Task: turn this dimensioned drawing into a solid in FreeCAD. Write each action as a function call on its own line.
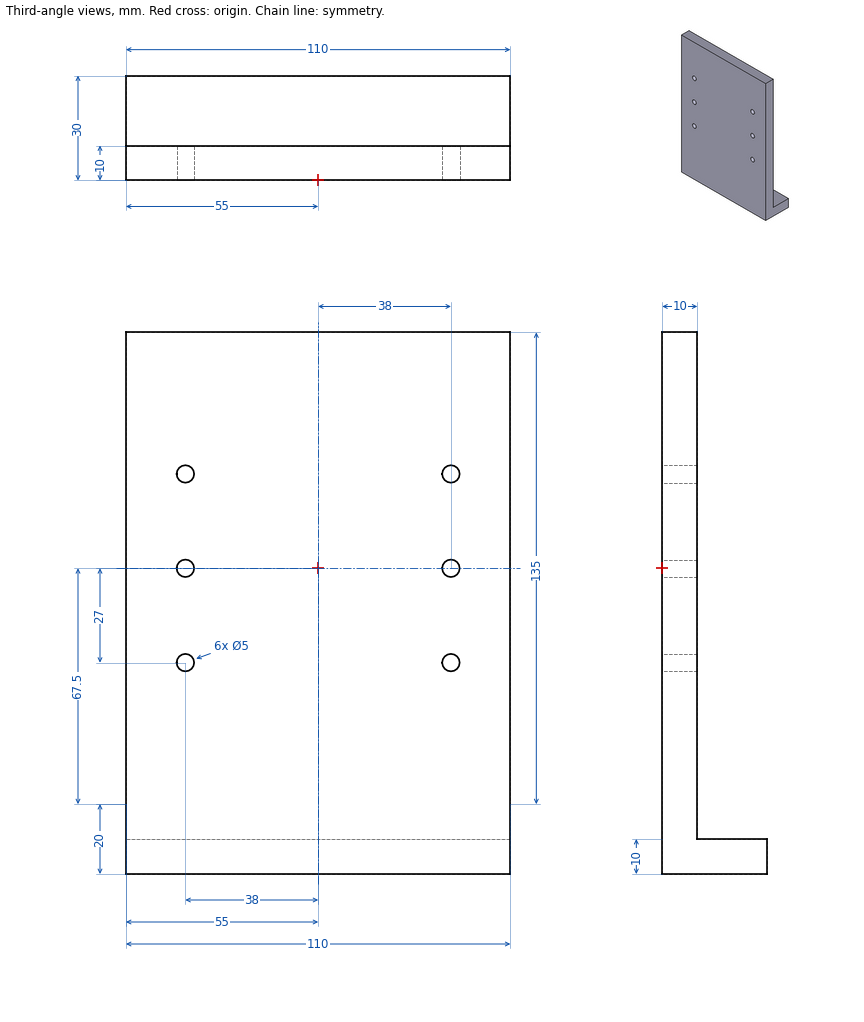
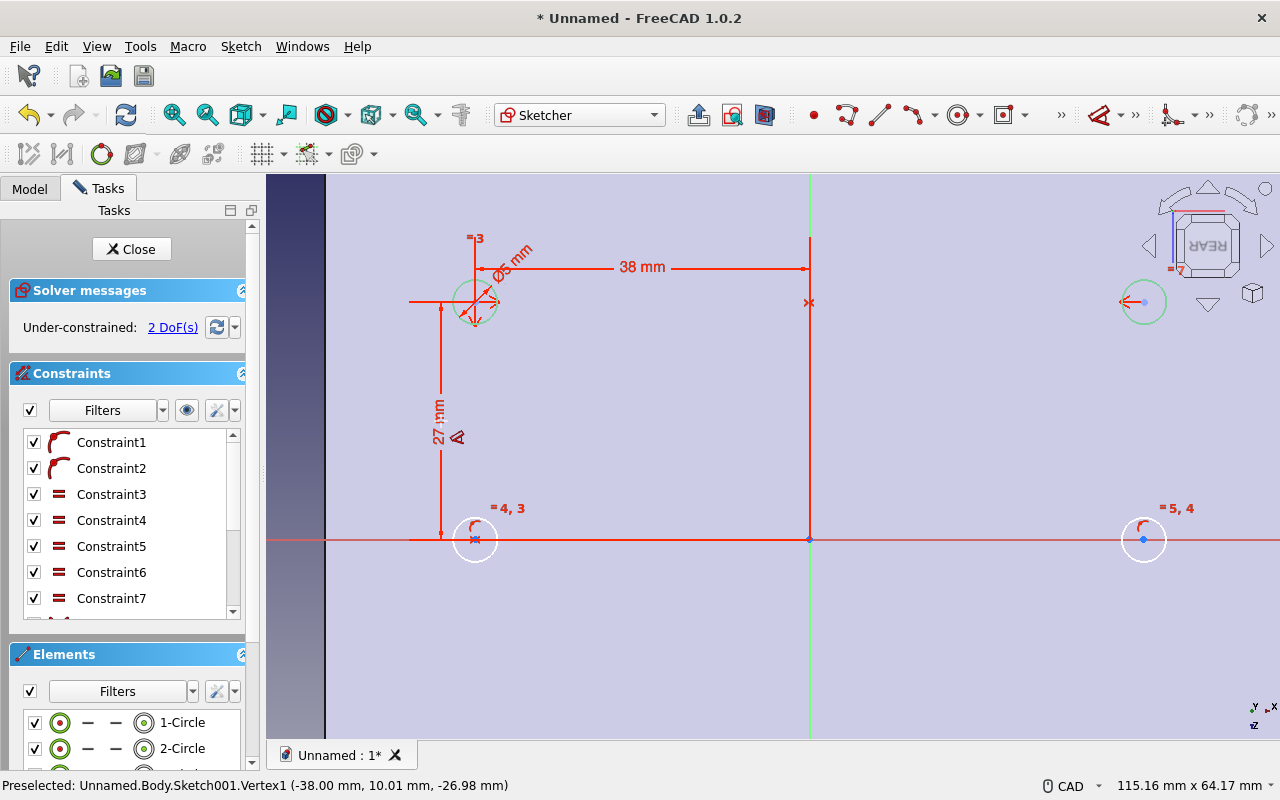
click(475, 540)
click(643, 574)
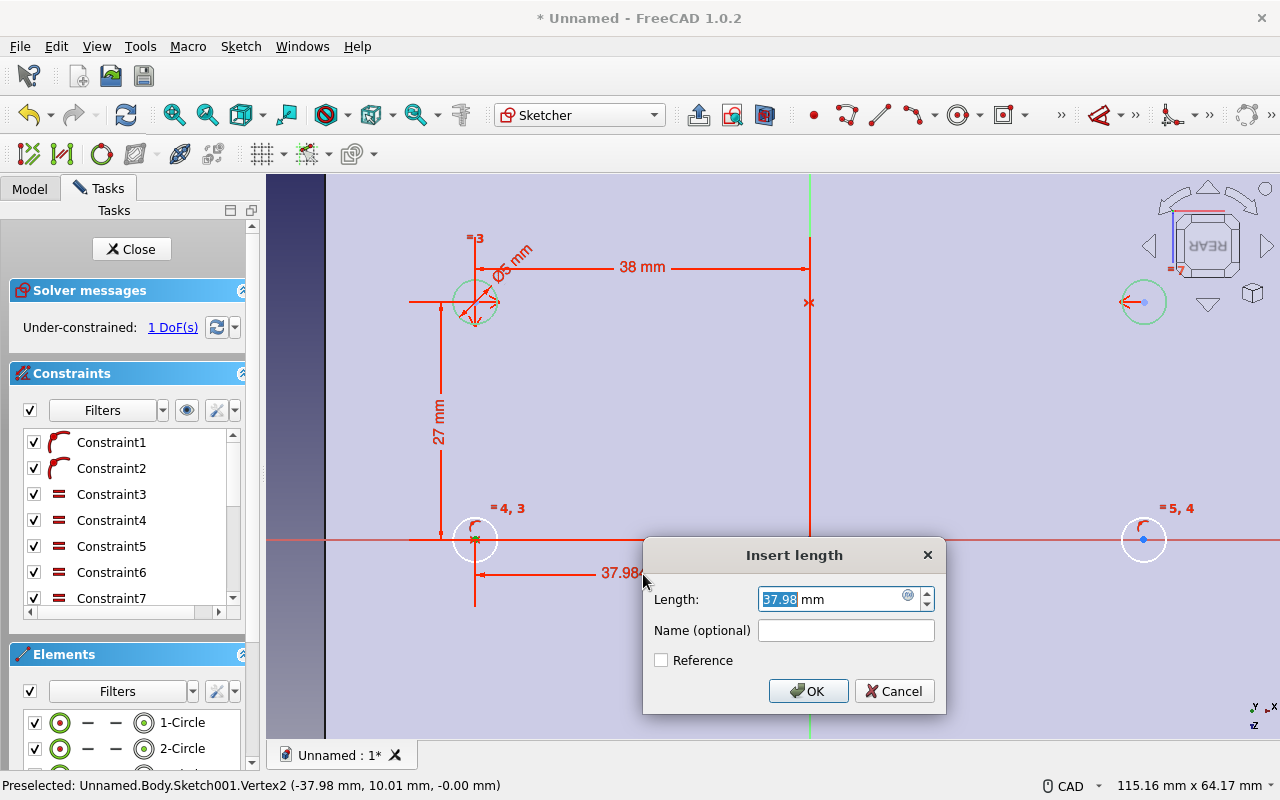
text(38)
key(Return)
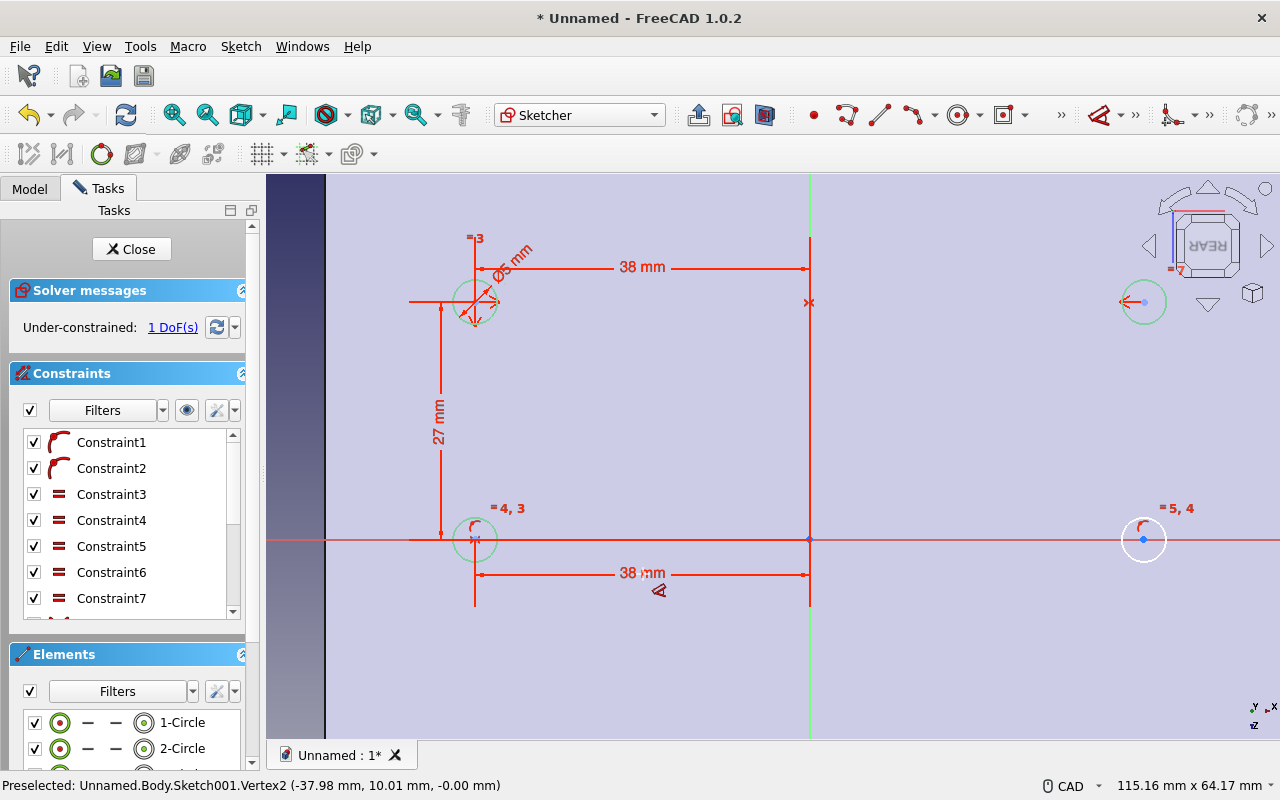
scroll(491, 287, down, 2)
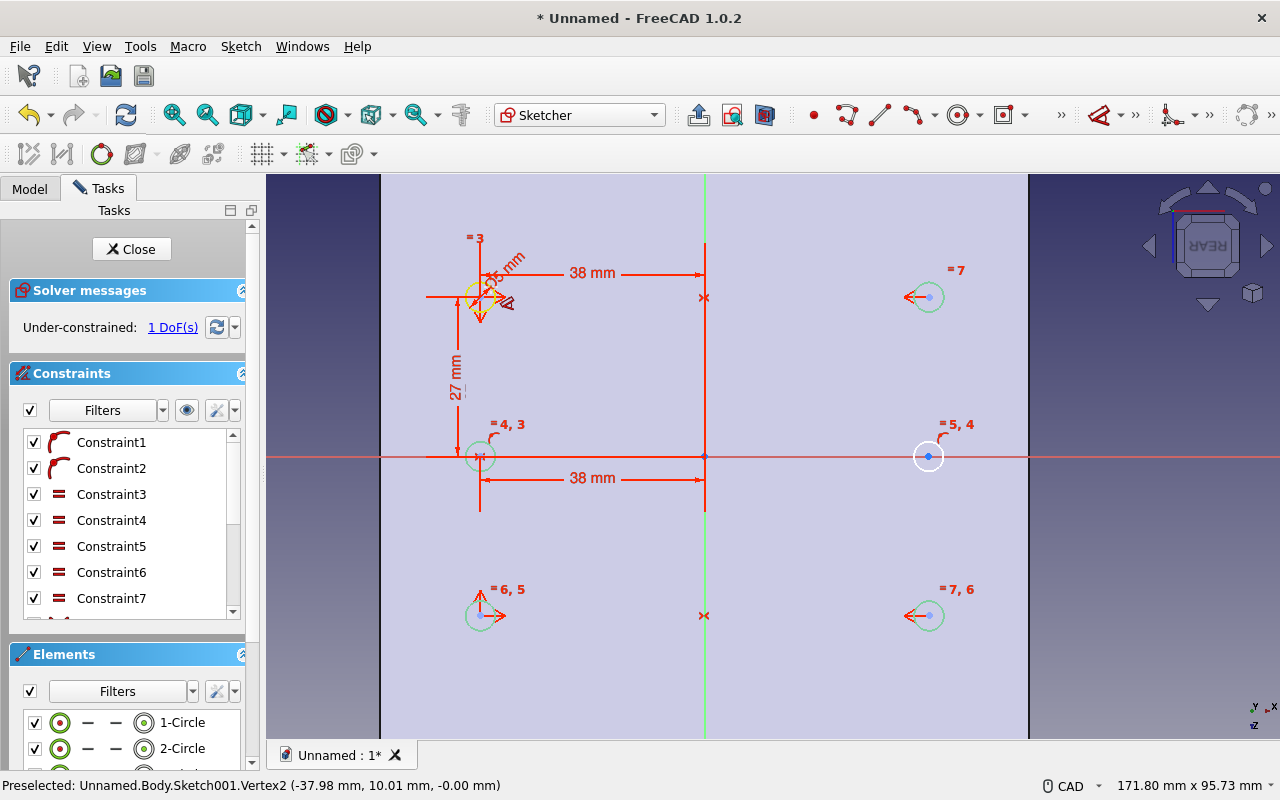
click(929, 457)
click(817, 491)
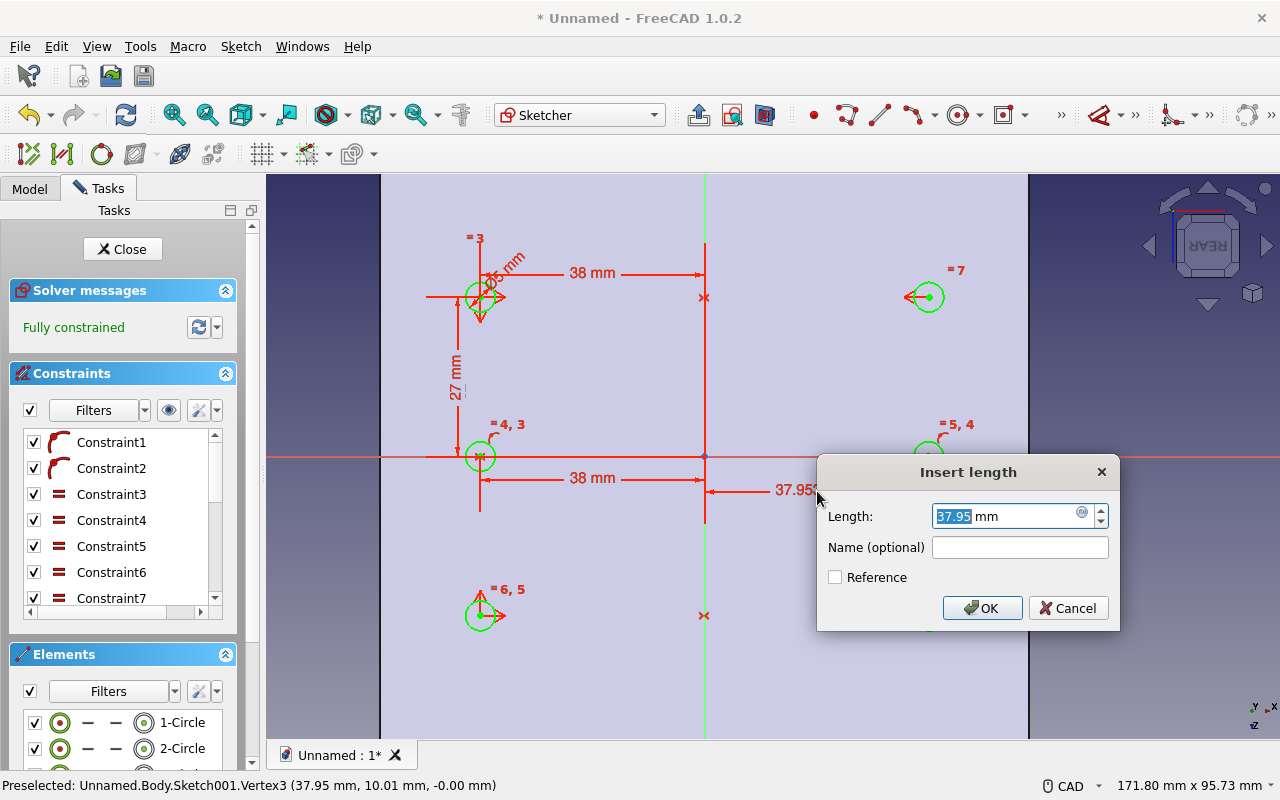
text(38)
key(Return)
key(Escape)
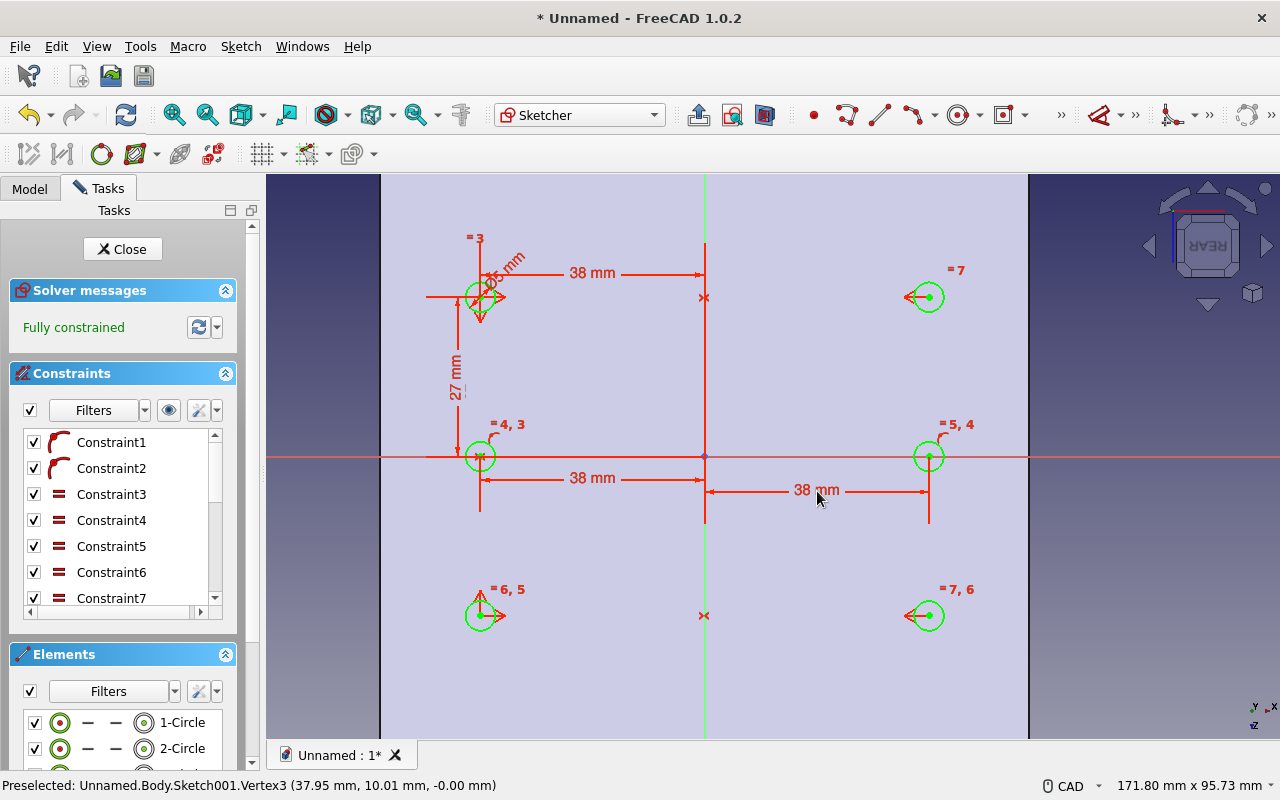
click(123, 249)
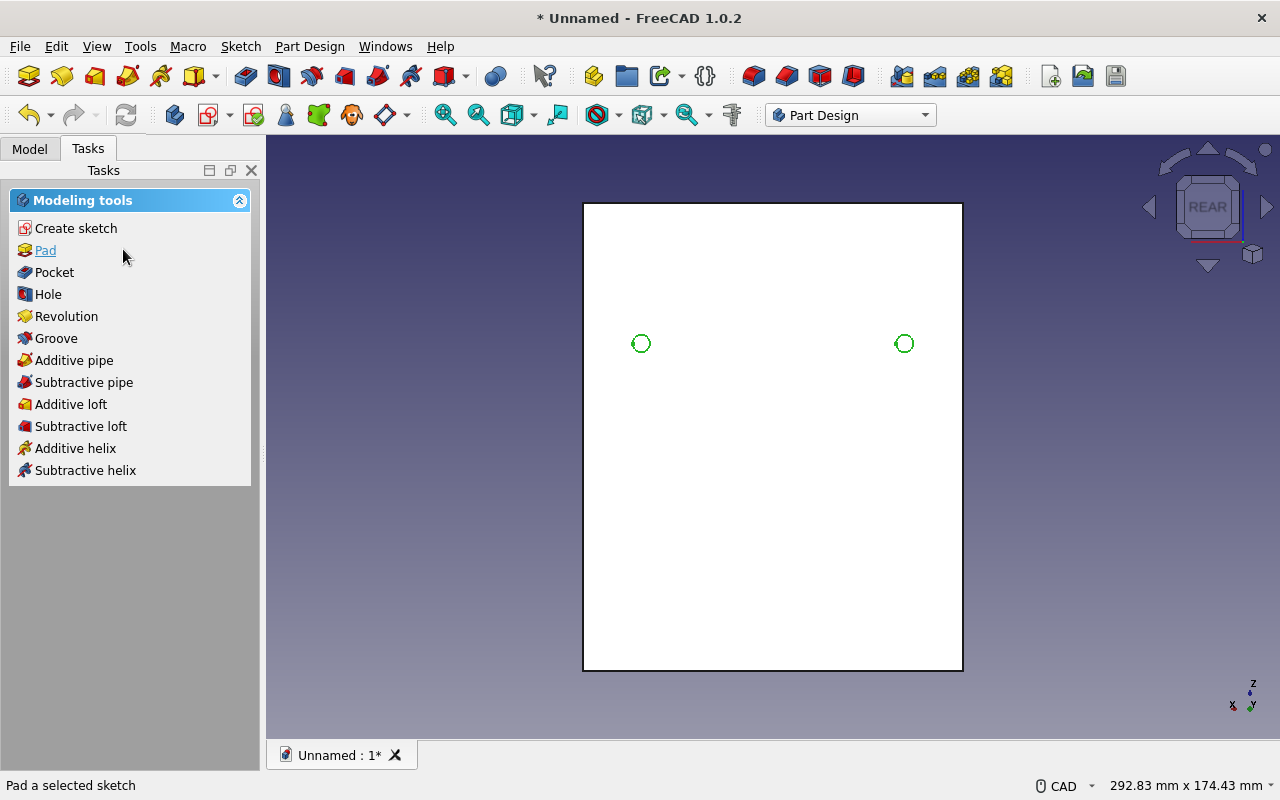
click(246, 76)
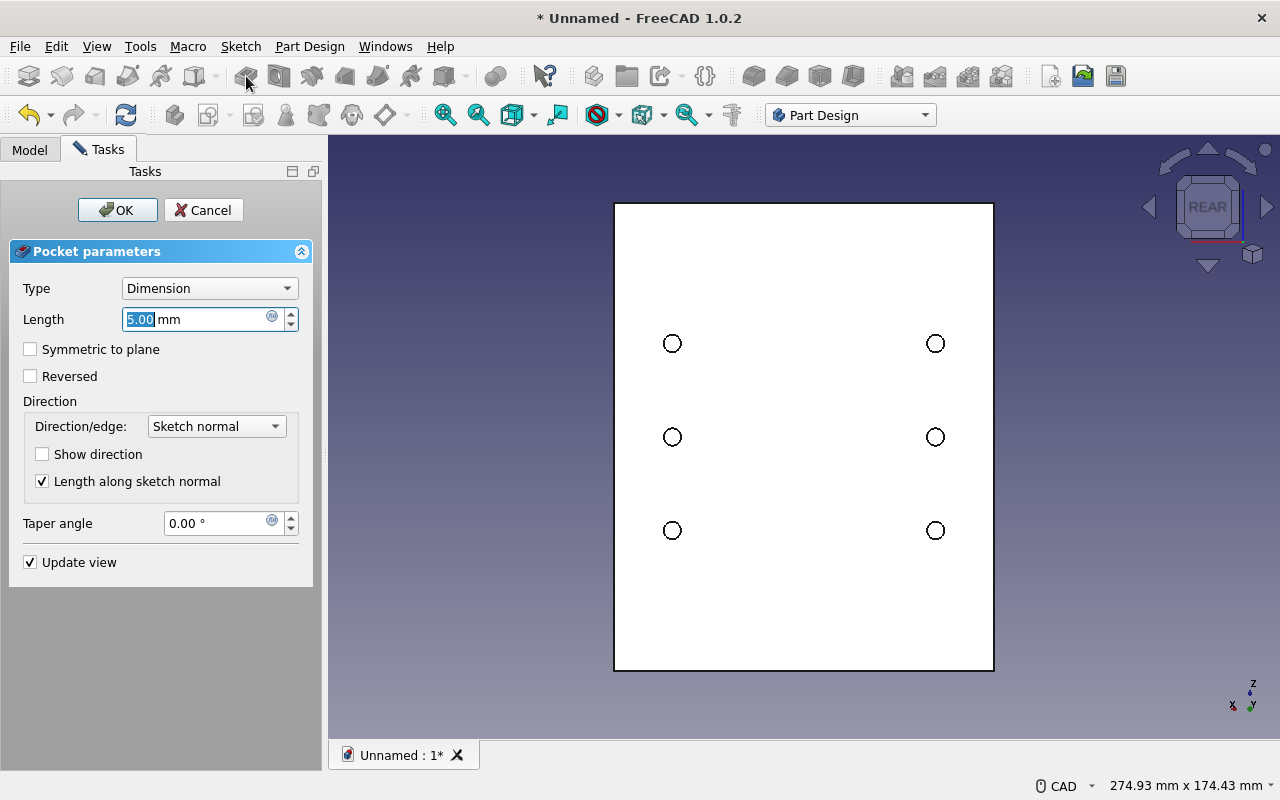
click(210, 288)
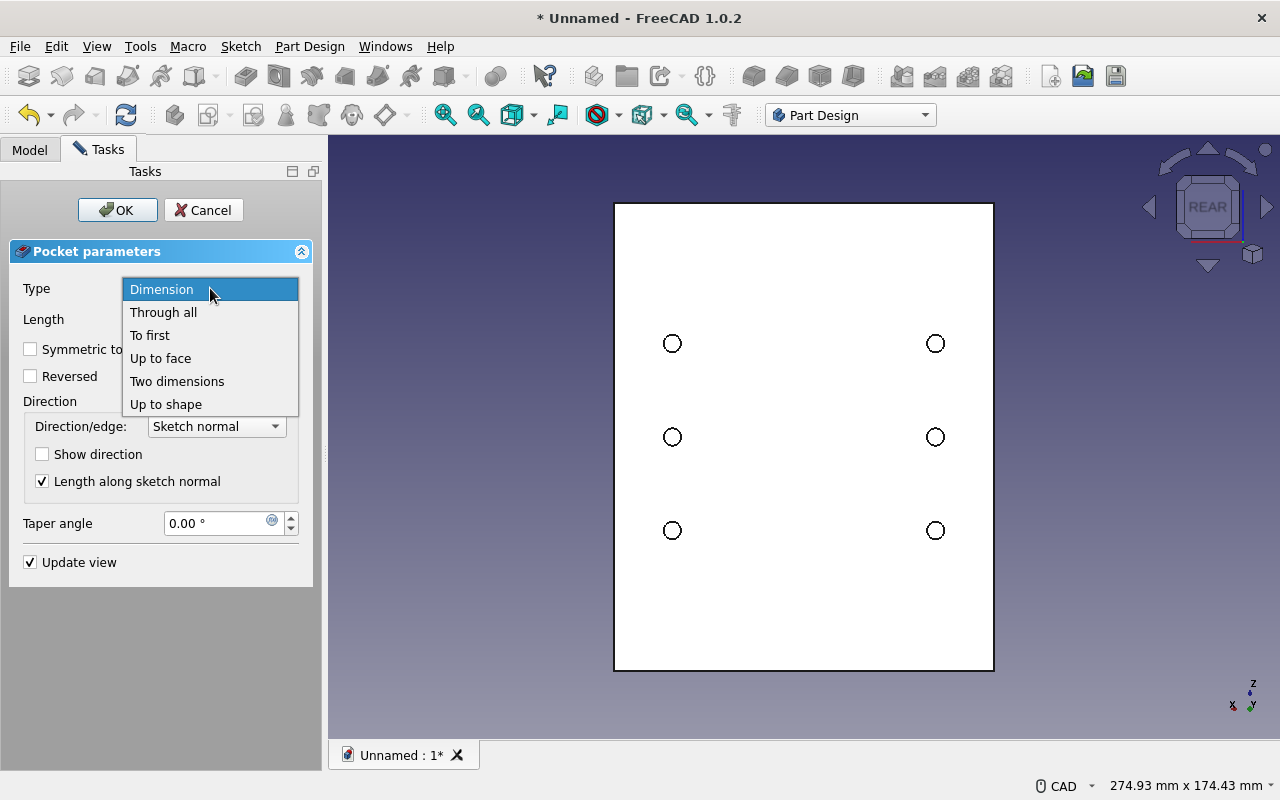
click(208, 312)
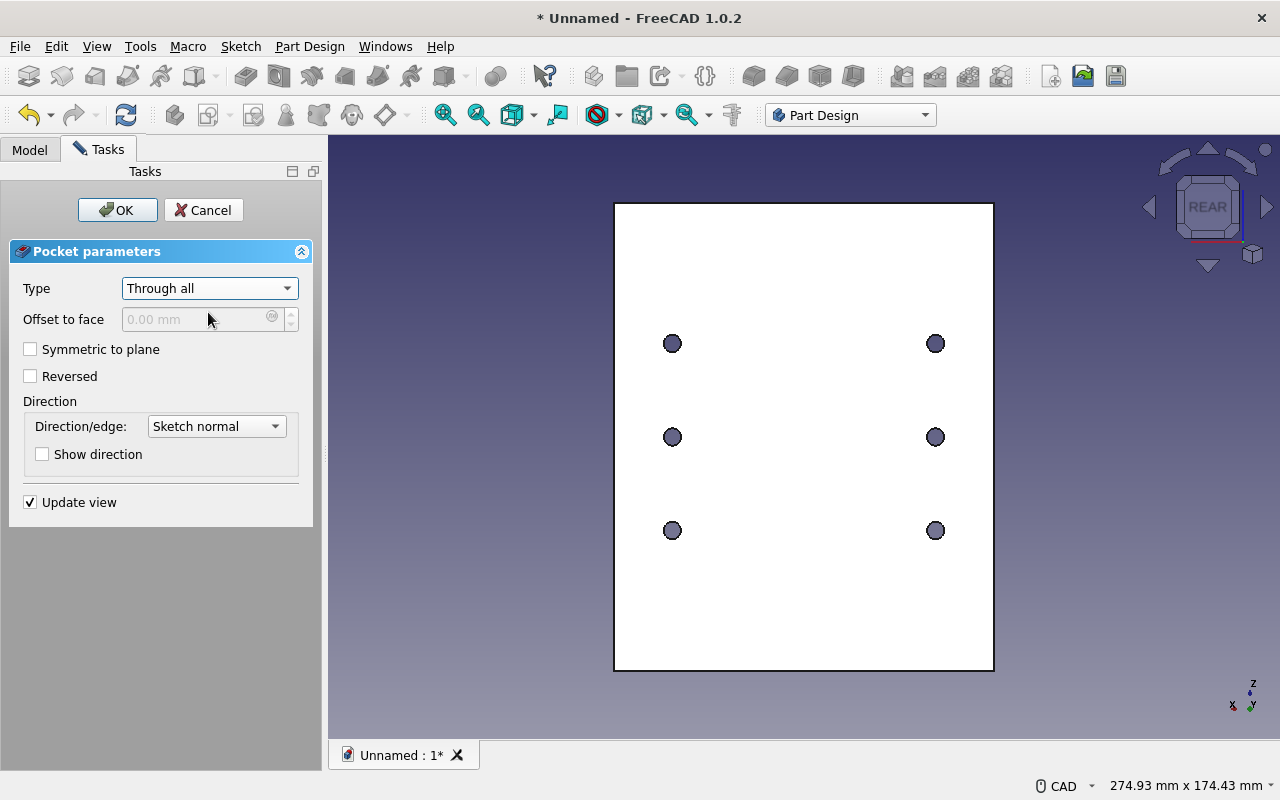
click(118, 210)